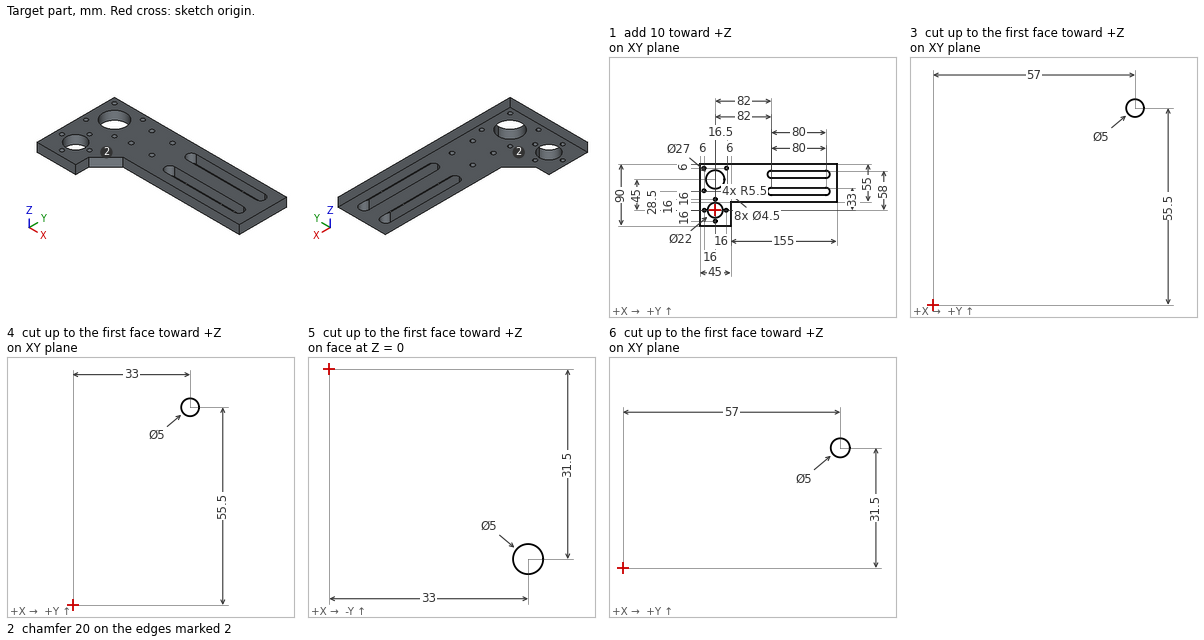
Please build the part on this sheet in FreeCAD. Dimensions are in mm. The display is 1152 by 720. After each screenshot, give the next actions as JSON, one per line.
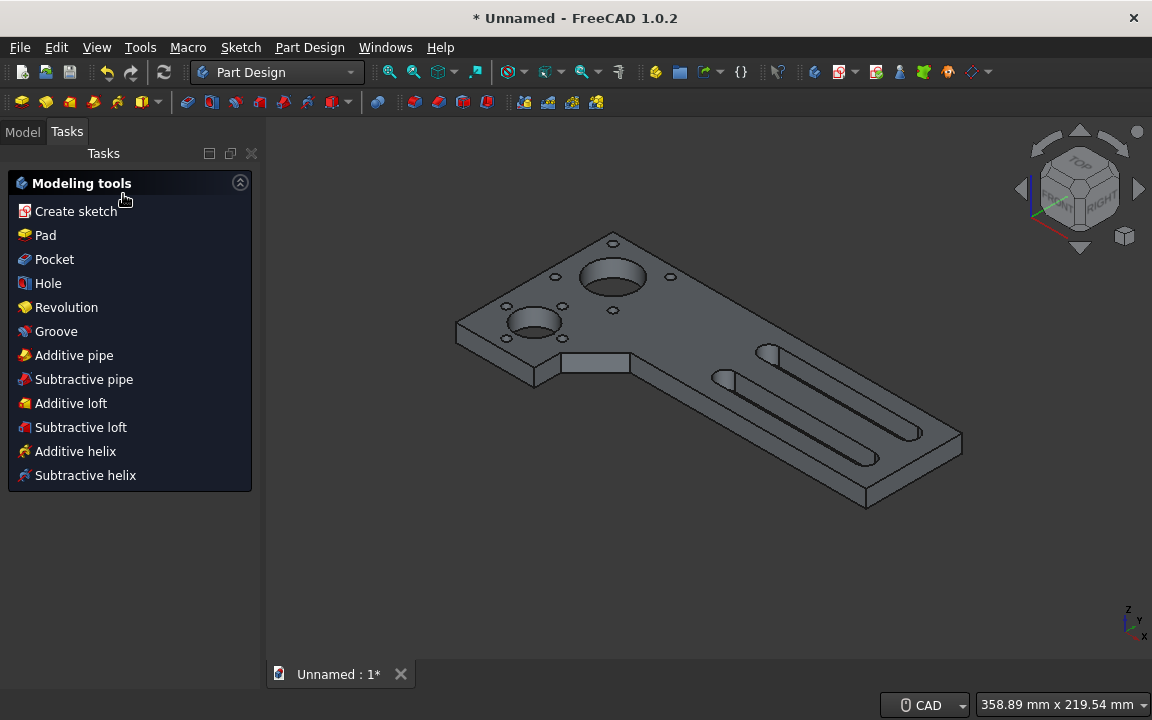
{"action": "left_click", "coordinate": [188, 102]}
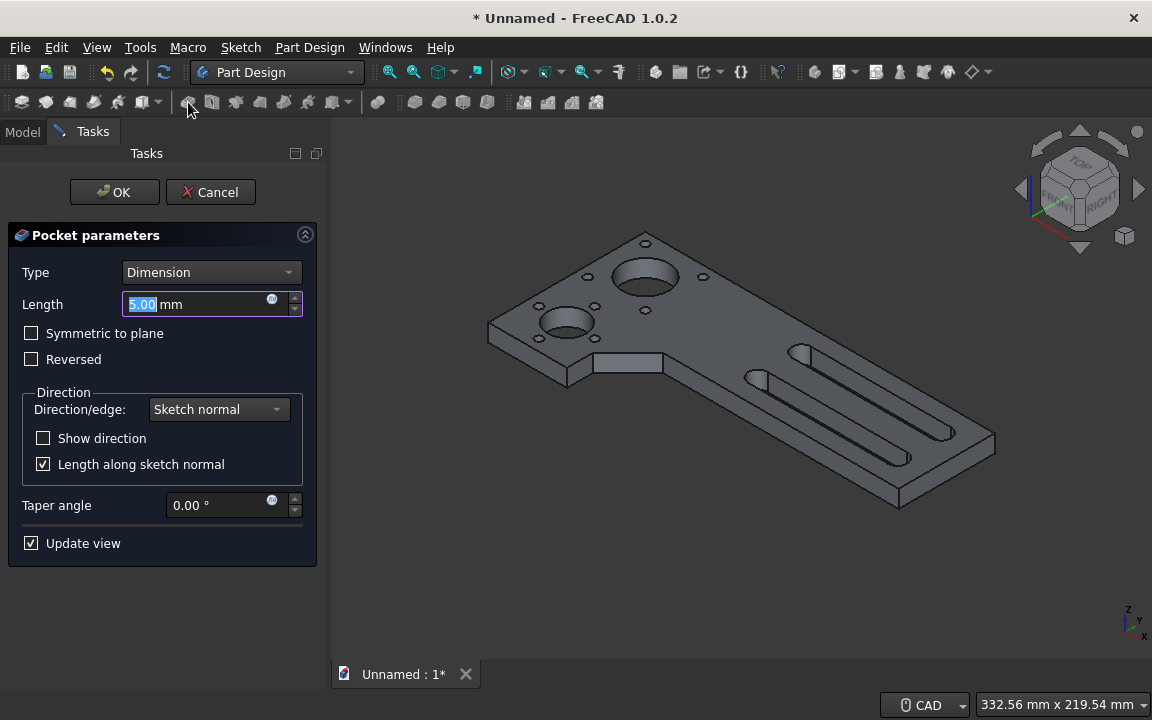
{"action": "left_click", "coordinate": [212, 272]}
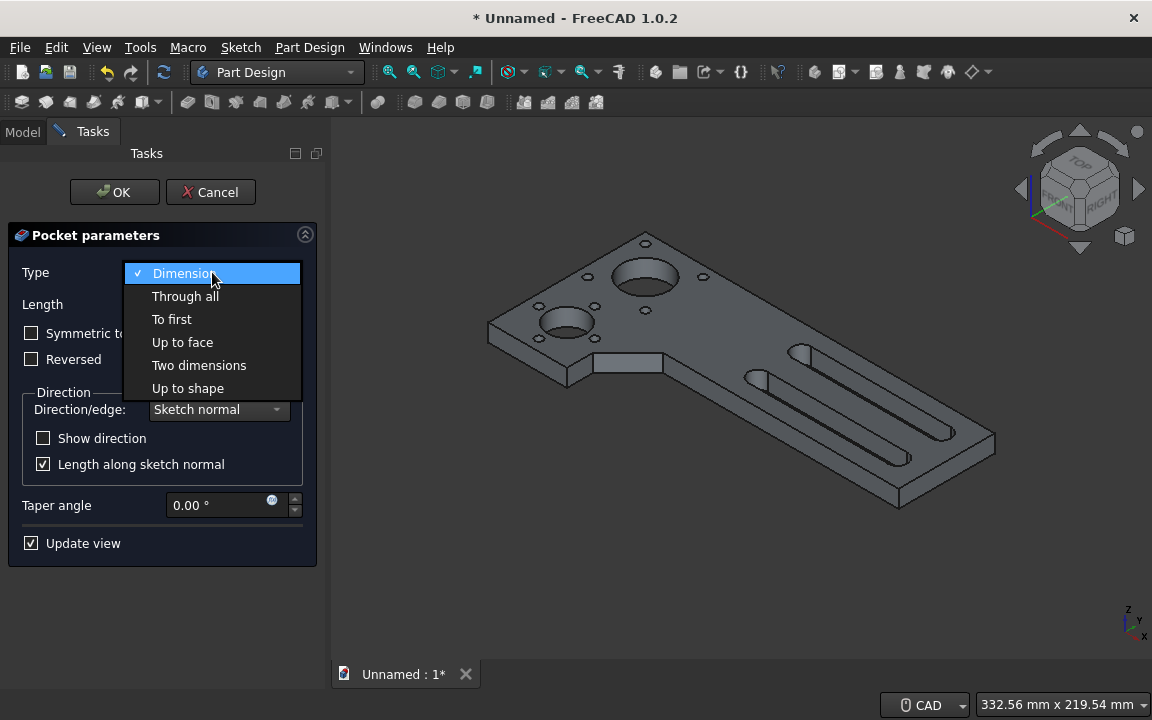
{"action": "left_click", "coordinate": [212, 320]}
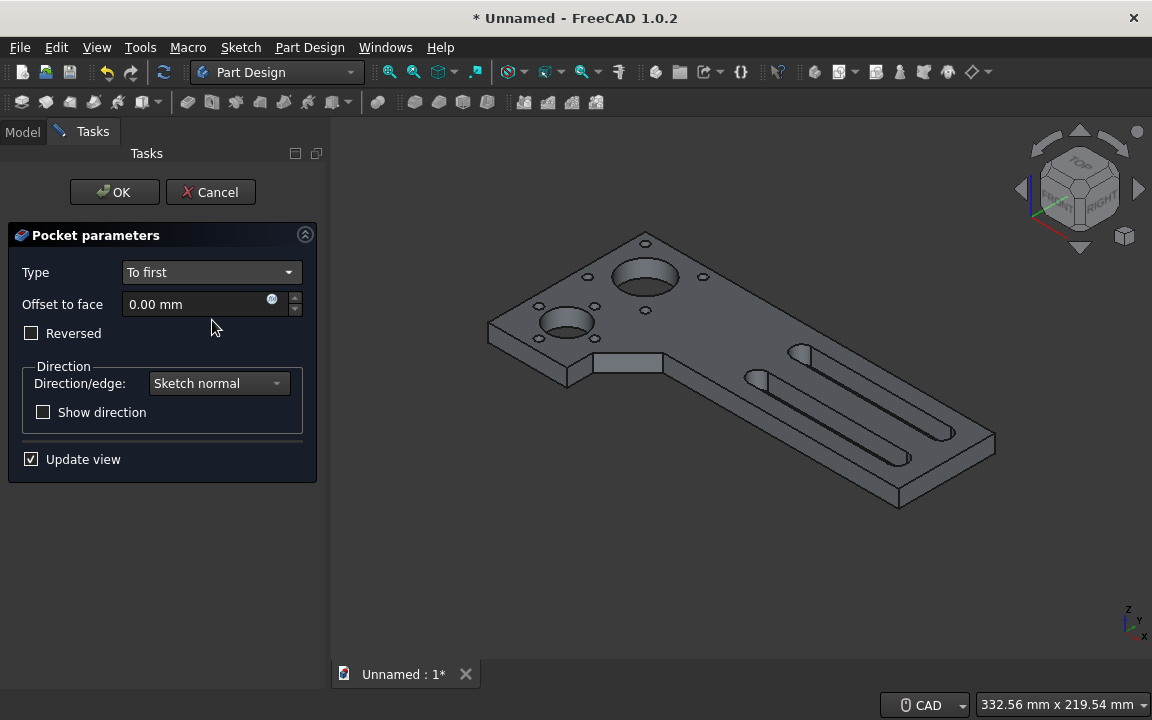
{"action": "left_click", "coordinate": [30, 333]}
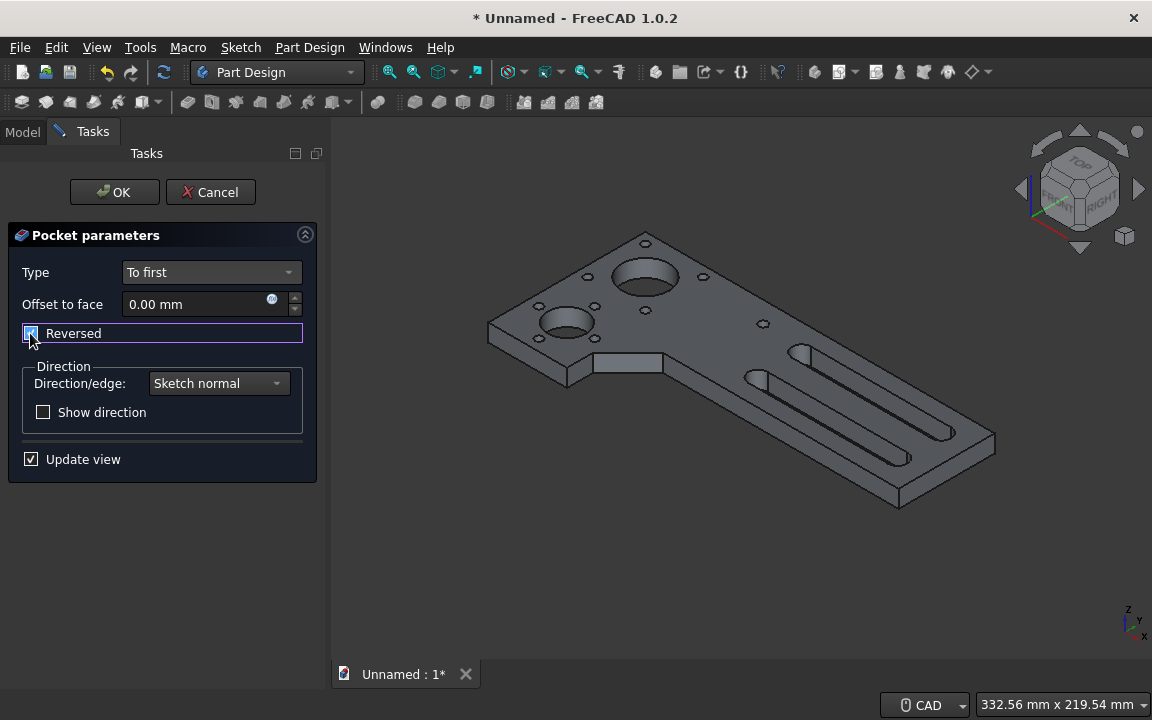
{"action": "left_click", "coordinate": [115, 192]}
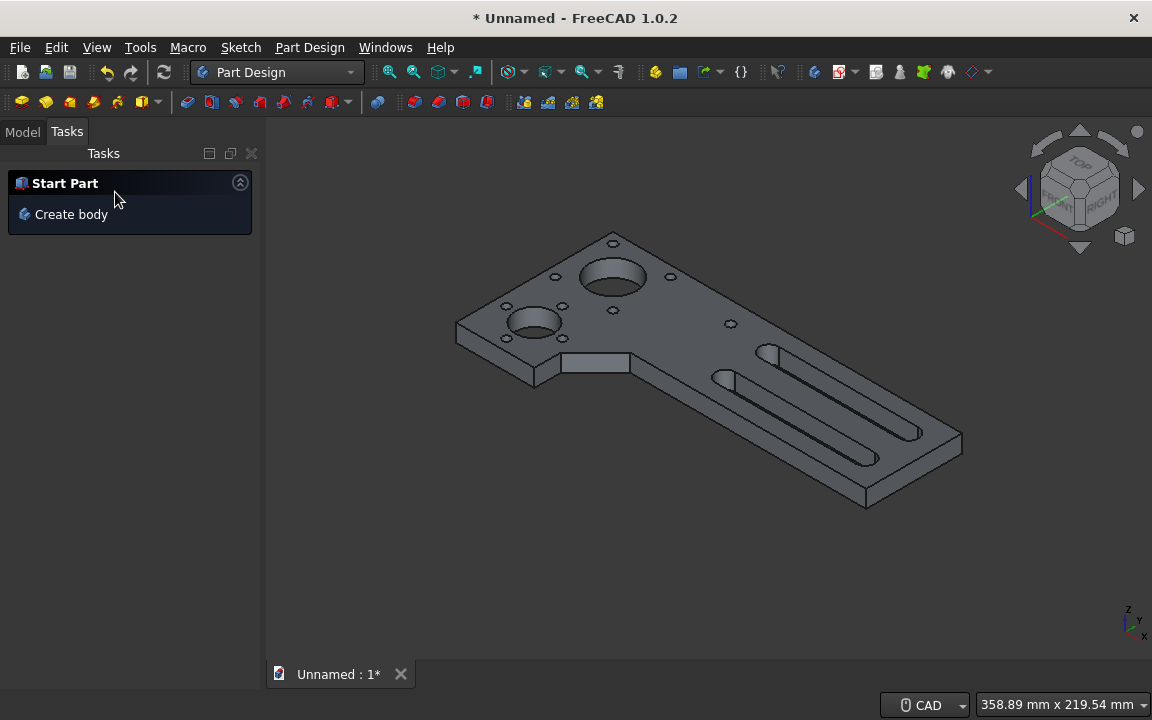
{"action": "left_click", "coordinate": [840, 72]}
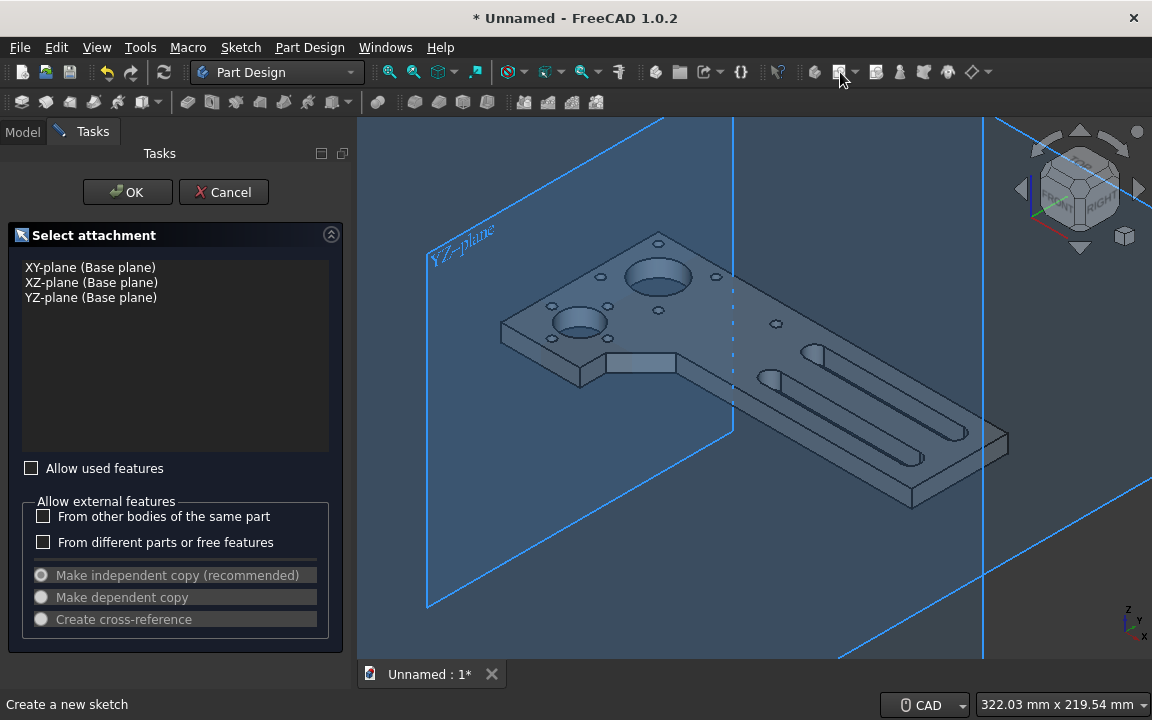
{"action": "left_click", "coordinate": [82, 268]}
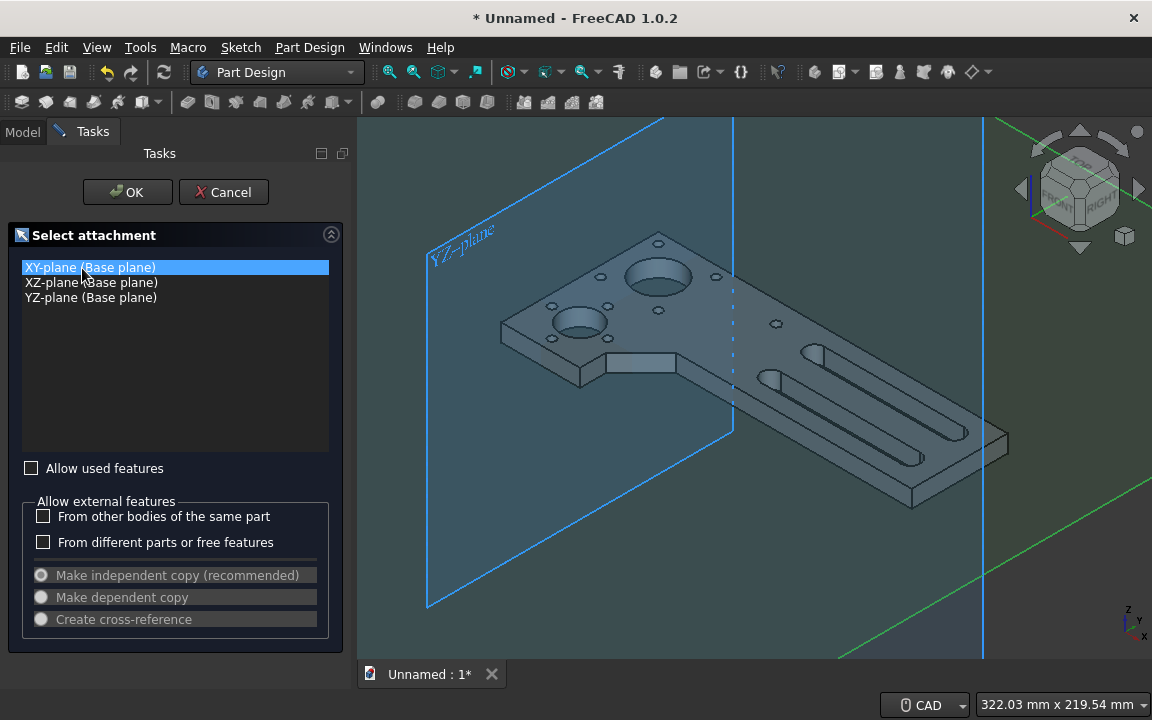
{"action": "left_click", "coordinate": [128, 192]}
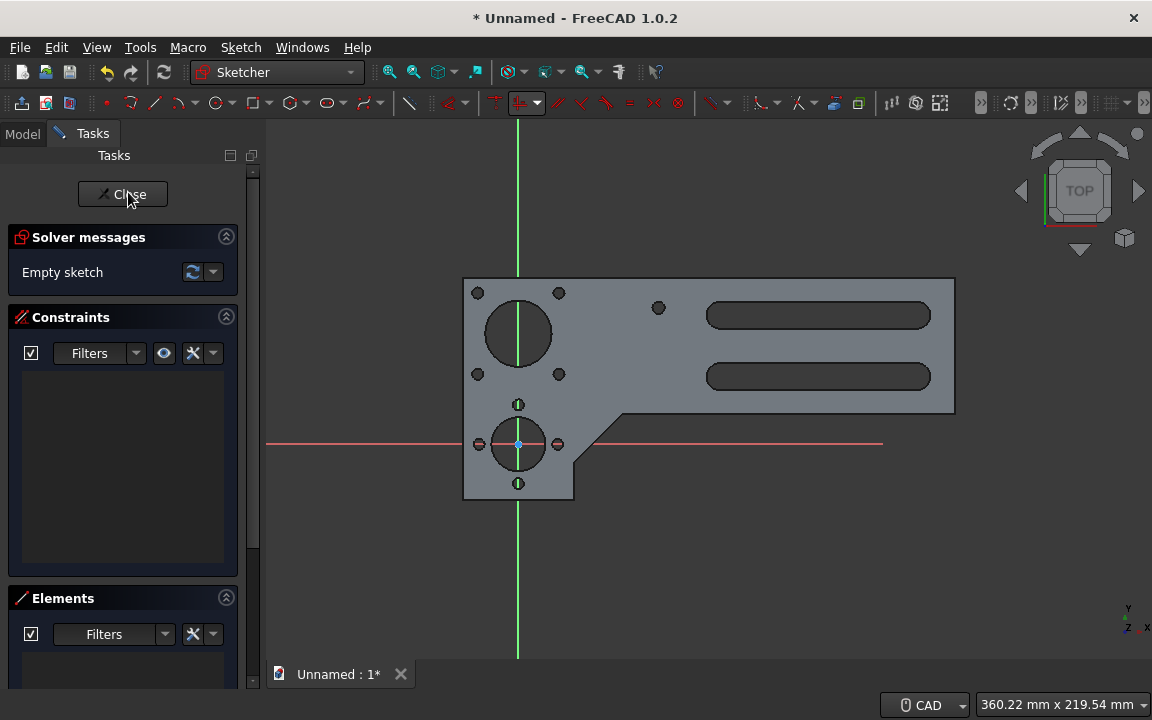
{"action": "key", "text": "q s"}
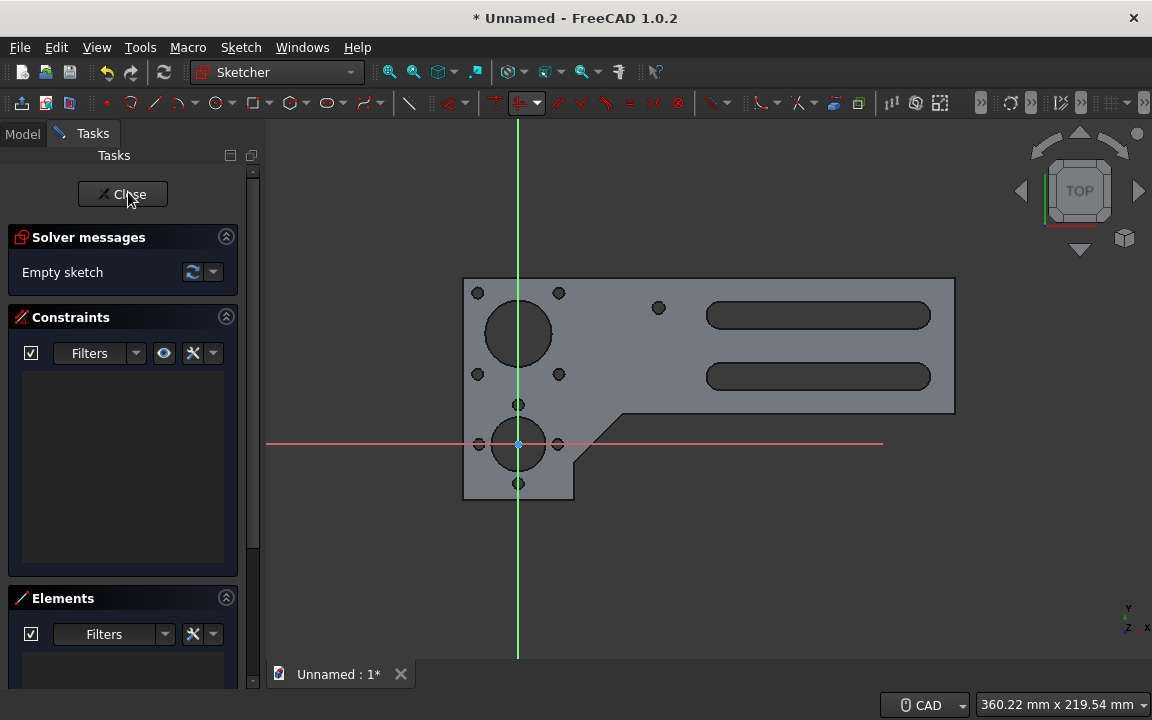
{"action": "scroll", "coordinate": [597, 304], "scroll_direction": "up", "scroll_amount": 15}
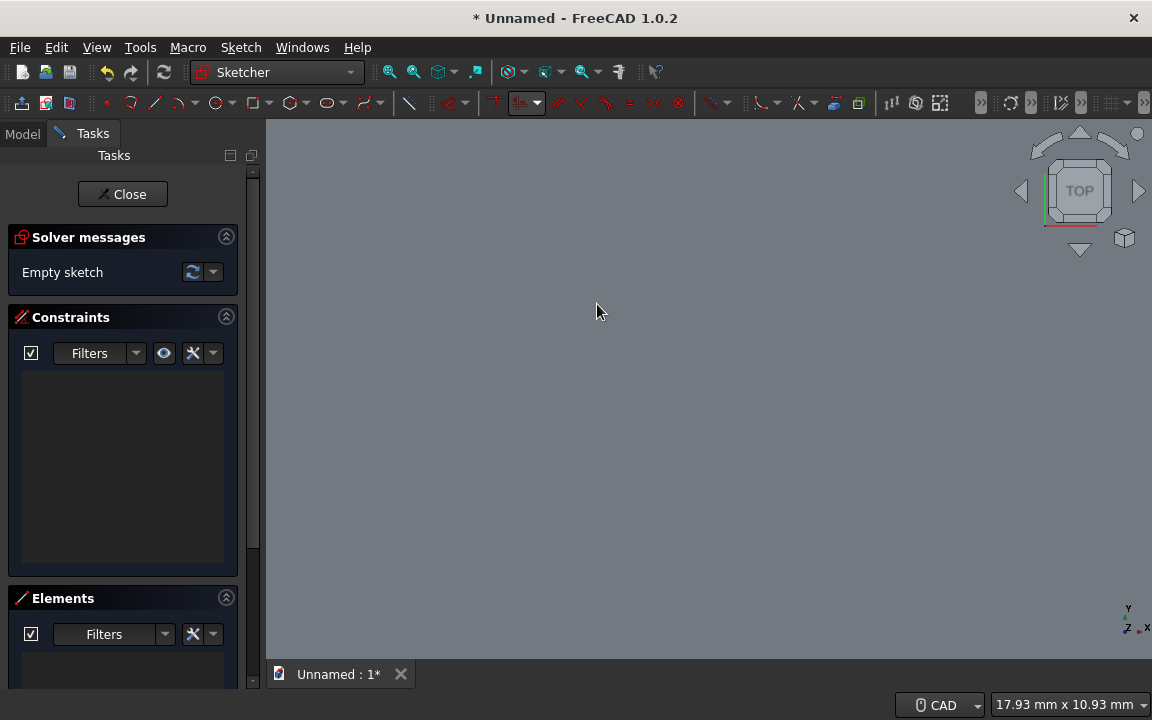
{"action": "scroll", "coordinate": [642, 345], "scroll_direction": "up", "scroll_amount": 2}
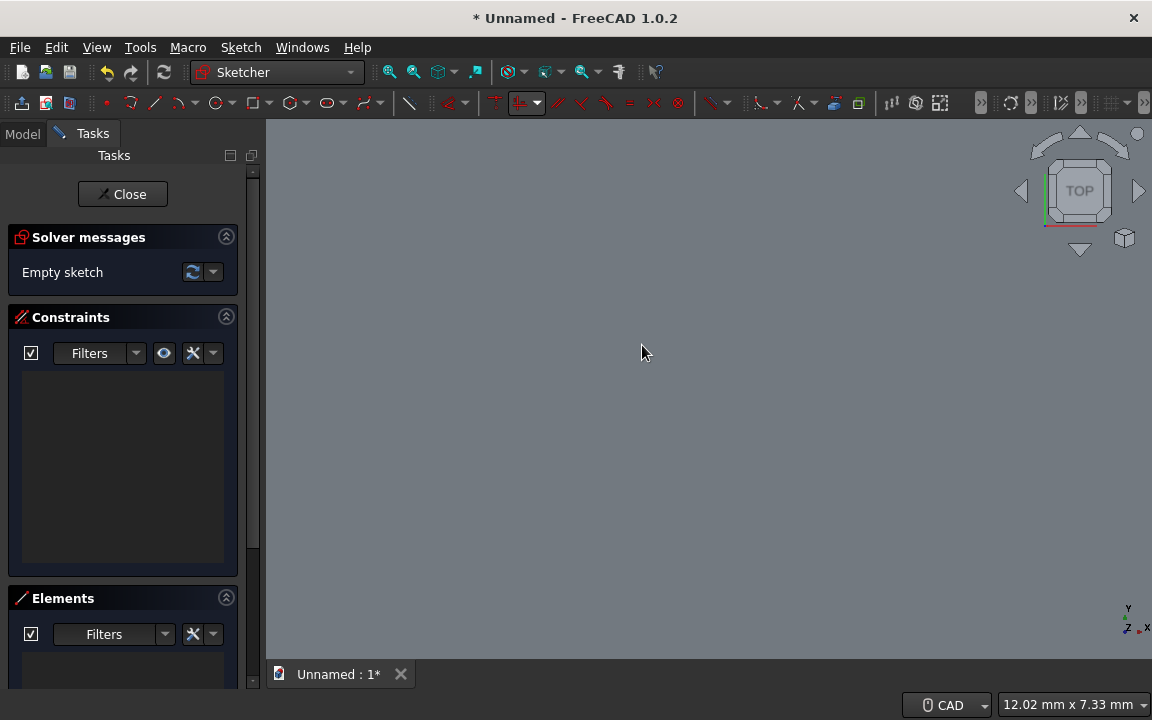
{"action": "key", "text": "g c"}